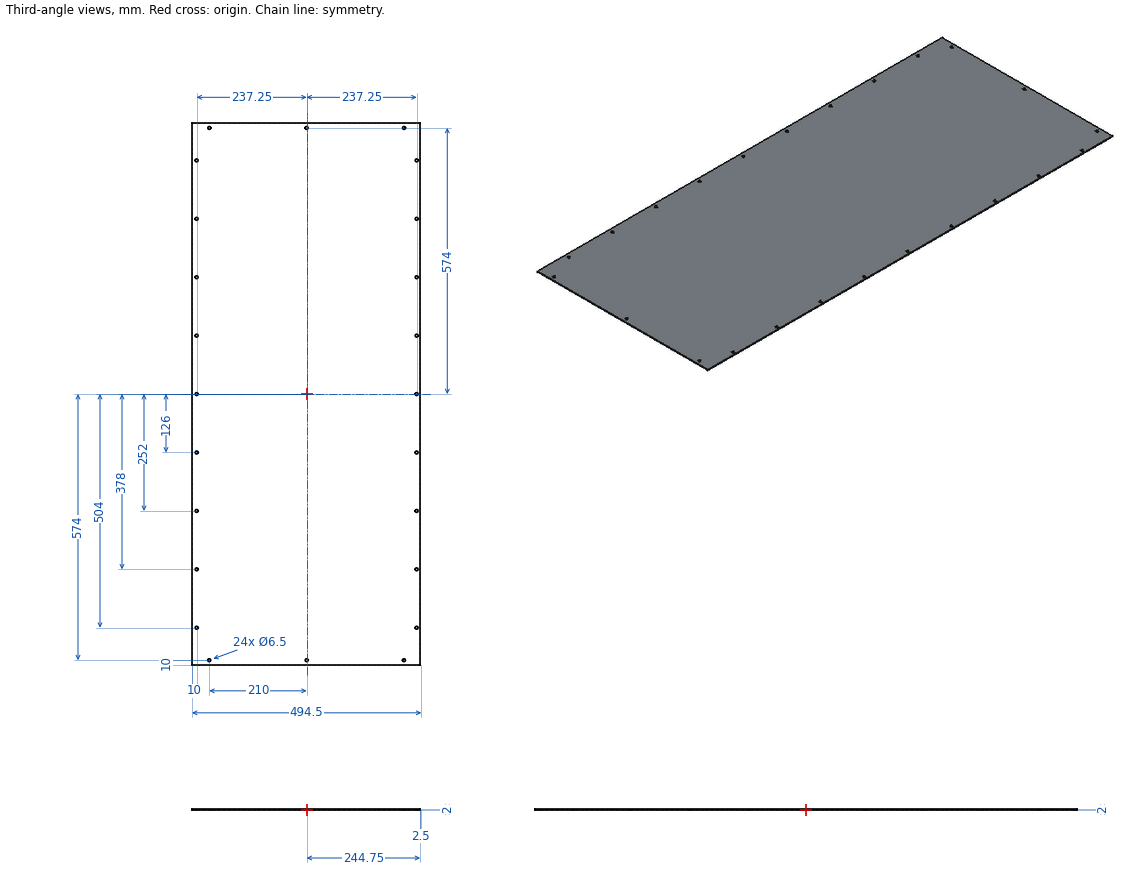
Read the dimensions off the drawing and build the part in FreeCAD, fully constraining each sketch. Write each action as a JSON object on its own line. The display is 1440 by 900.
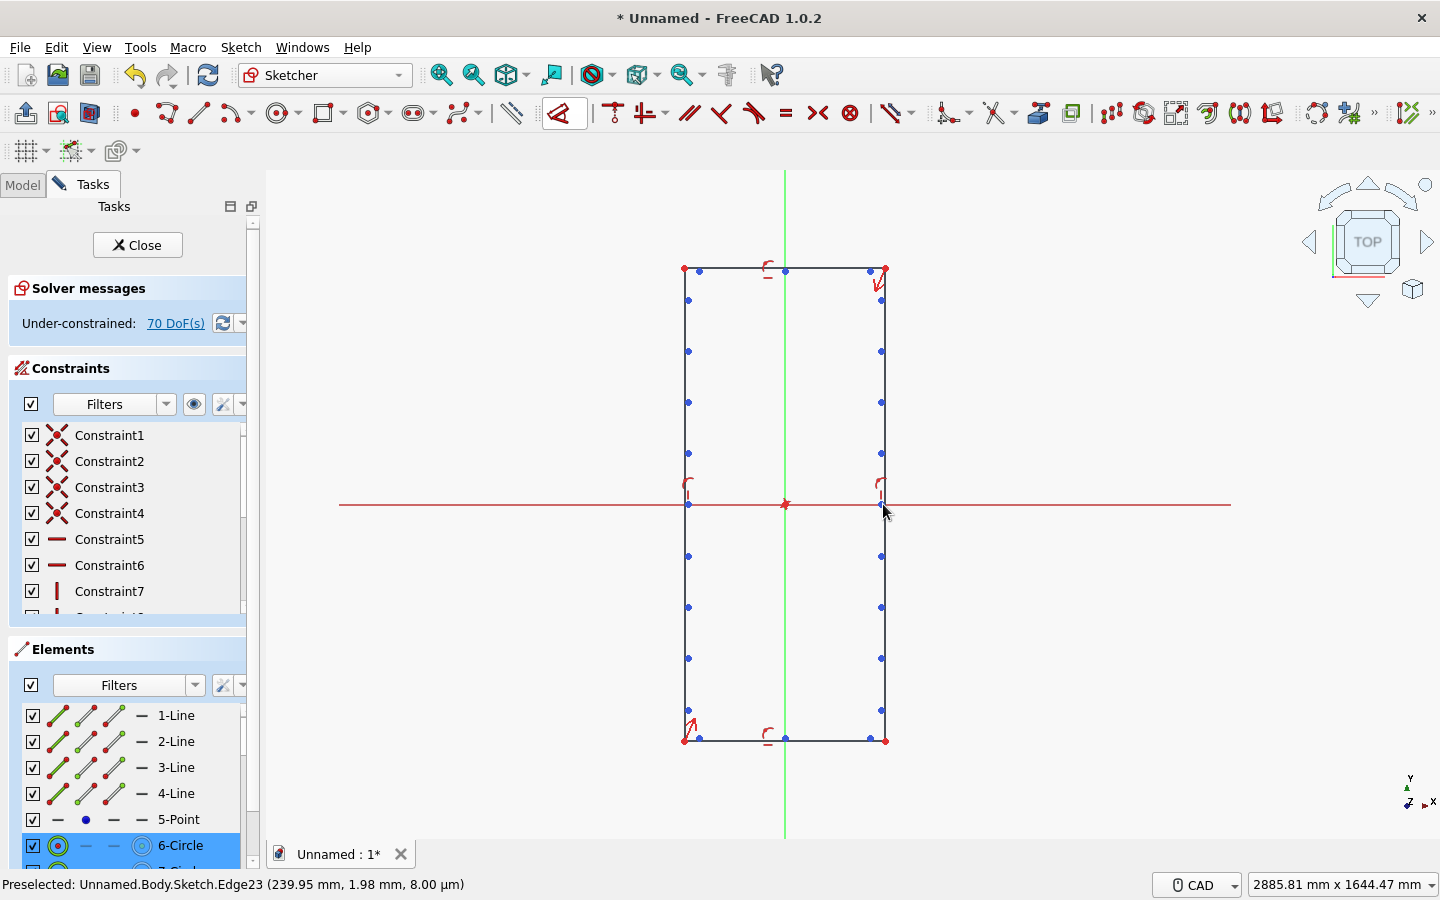
{"action": "scroll", "coordinate": [883, 453], "scroll_direction": "up", "scroll_amount": 12}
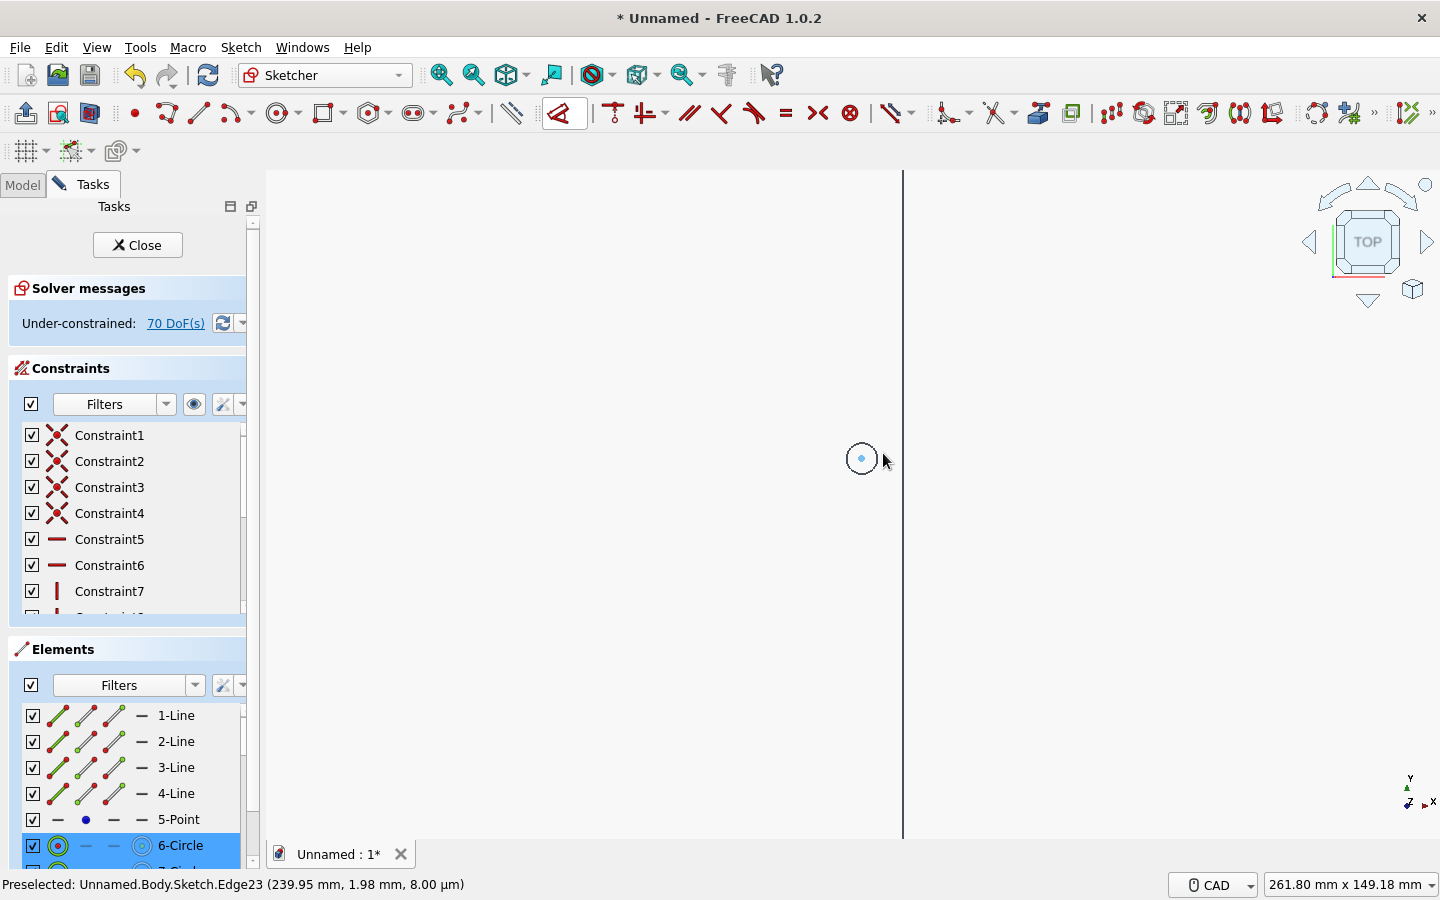
{"action": "left_click", "coordinate": [873, 448]}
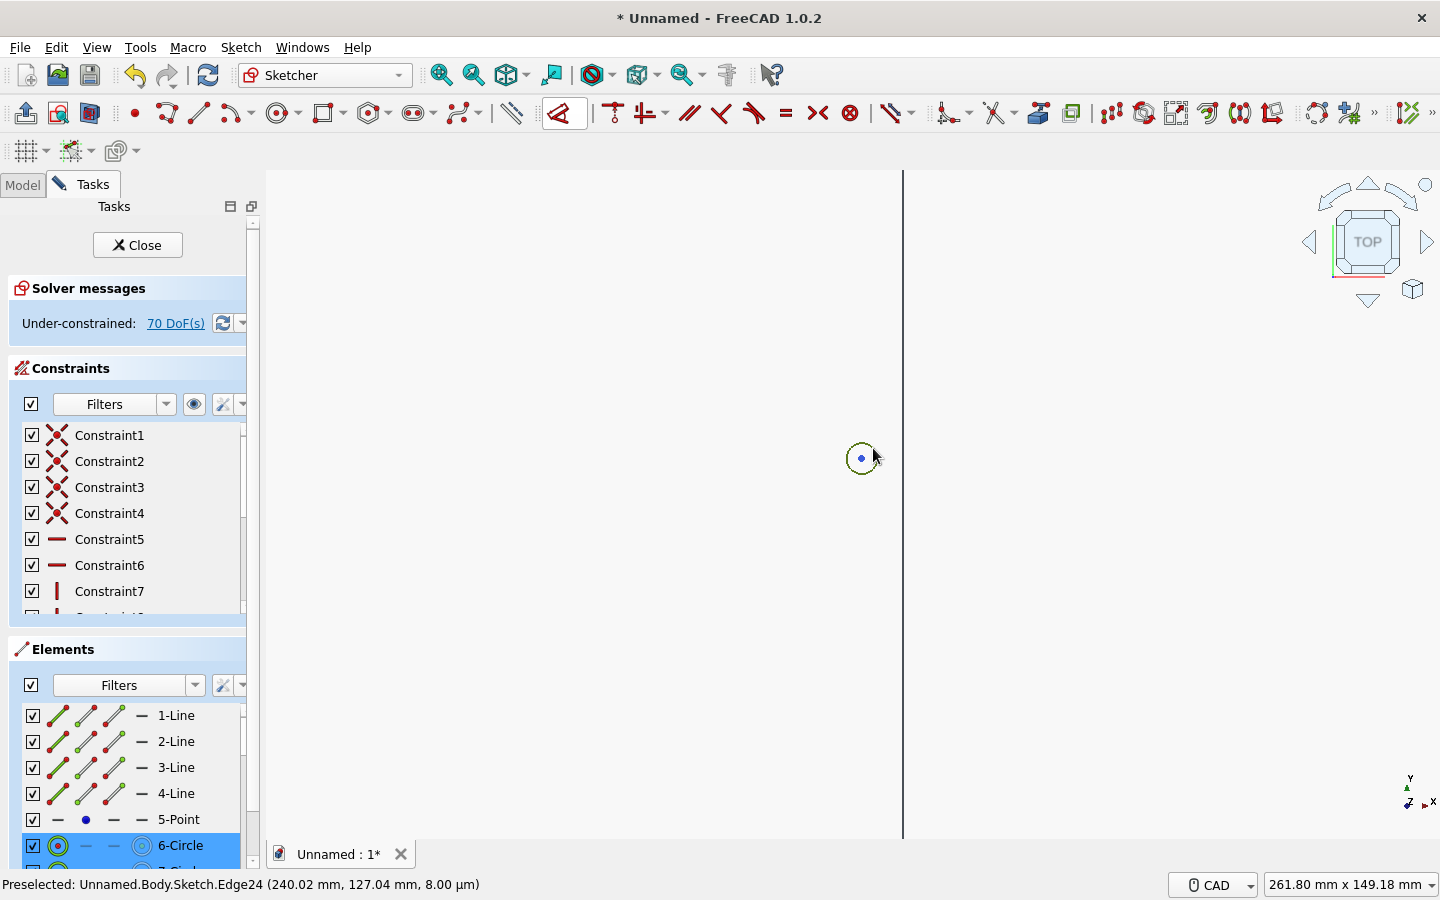
{"action": "scroll", "coordinate": [883, 453], "scroll_direction": "down", "scroll_amount": 12}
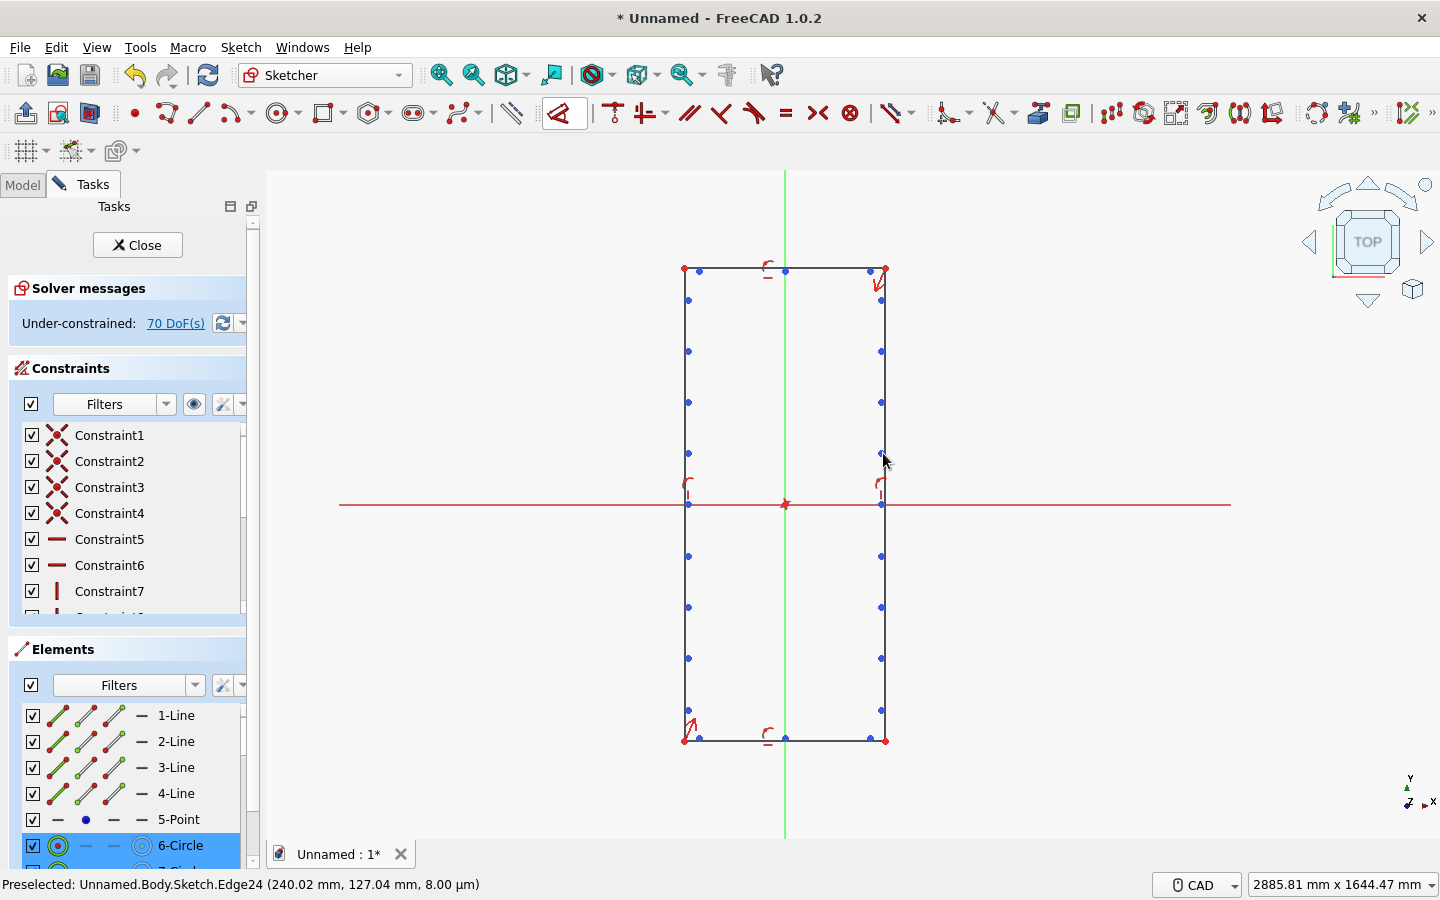
{"action": "scroll", "coordinate": [883, 402], "scroll_direction": "up", "scroll_amount": 12}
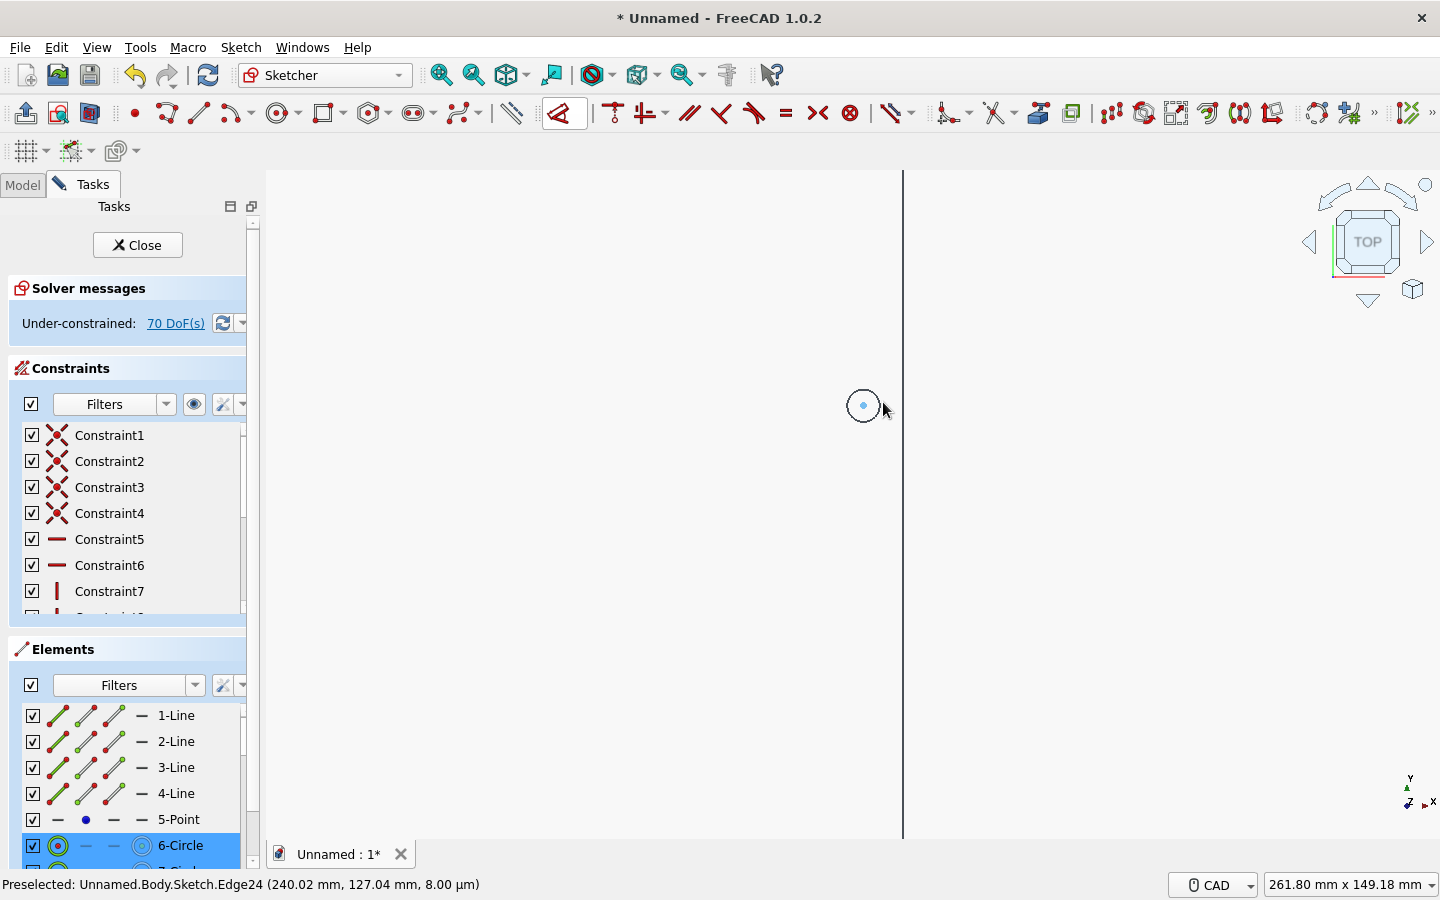
{"action": "left_click", "coordinate": [875, 394]}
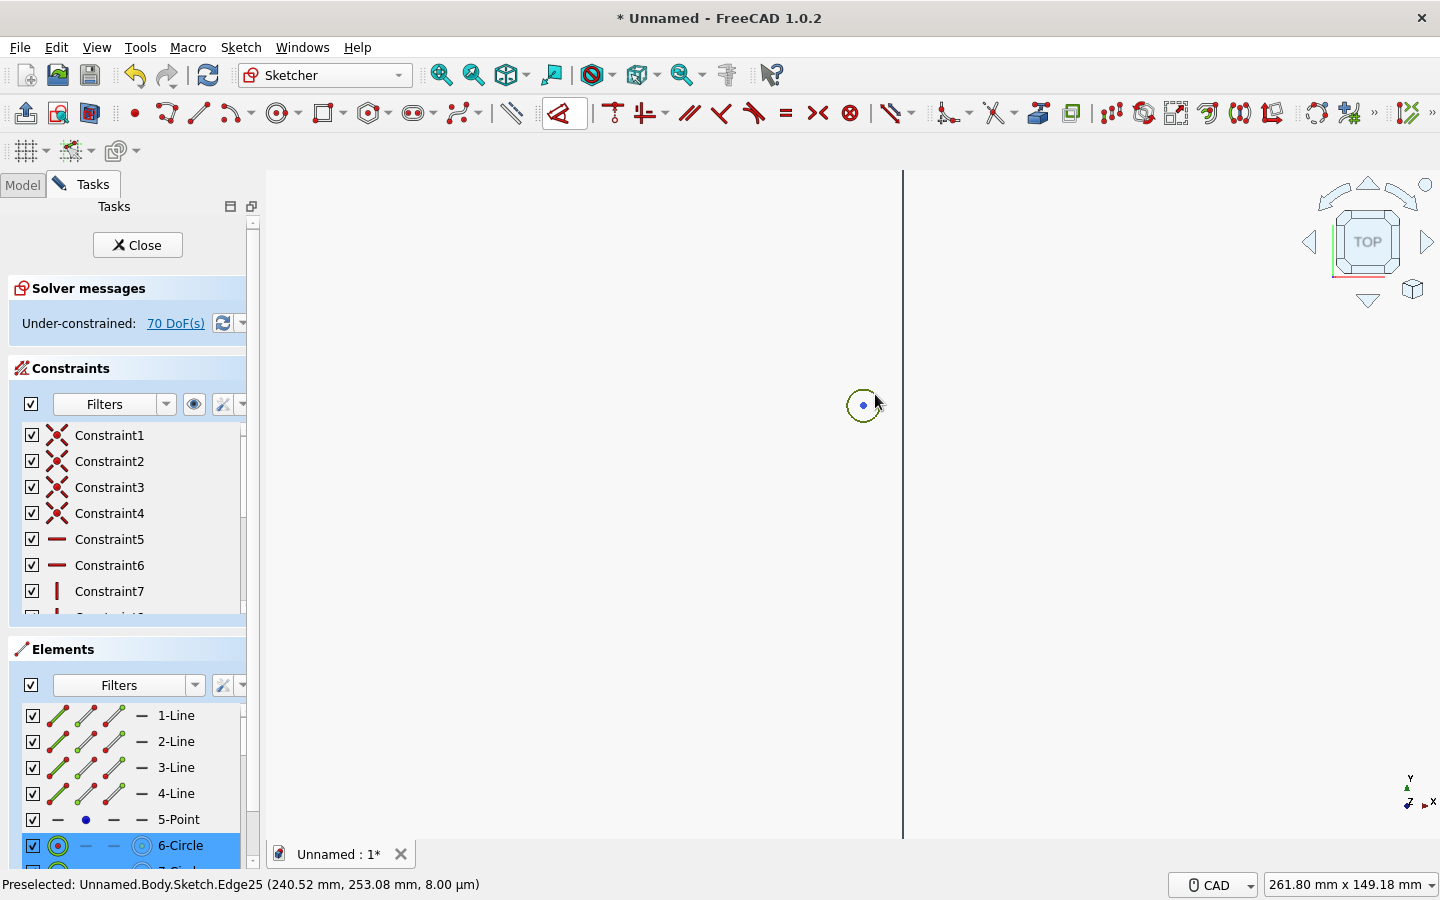
{"action": "scroll", "coordinate": [883, 402], "scroll_direction": "down", "scroll_amount": 12}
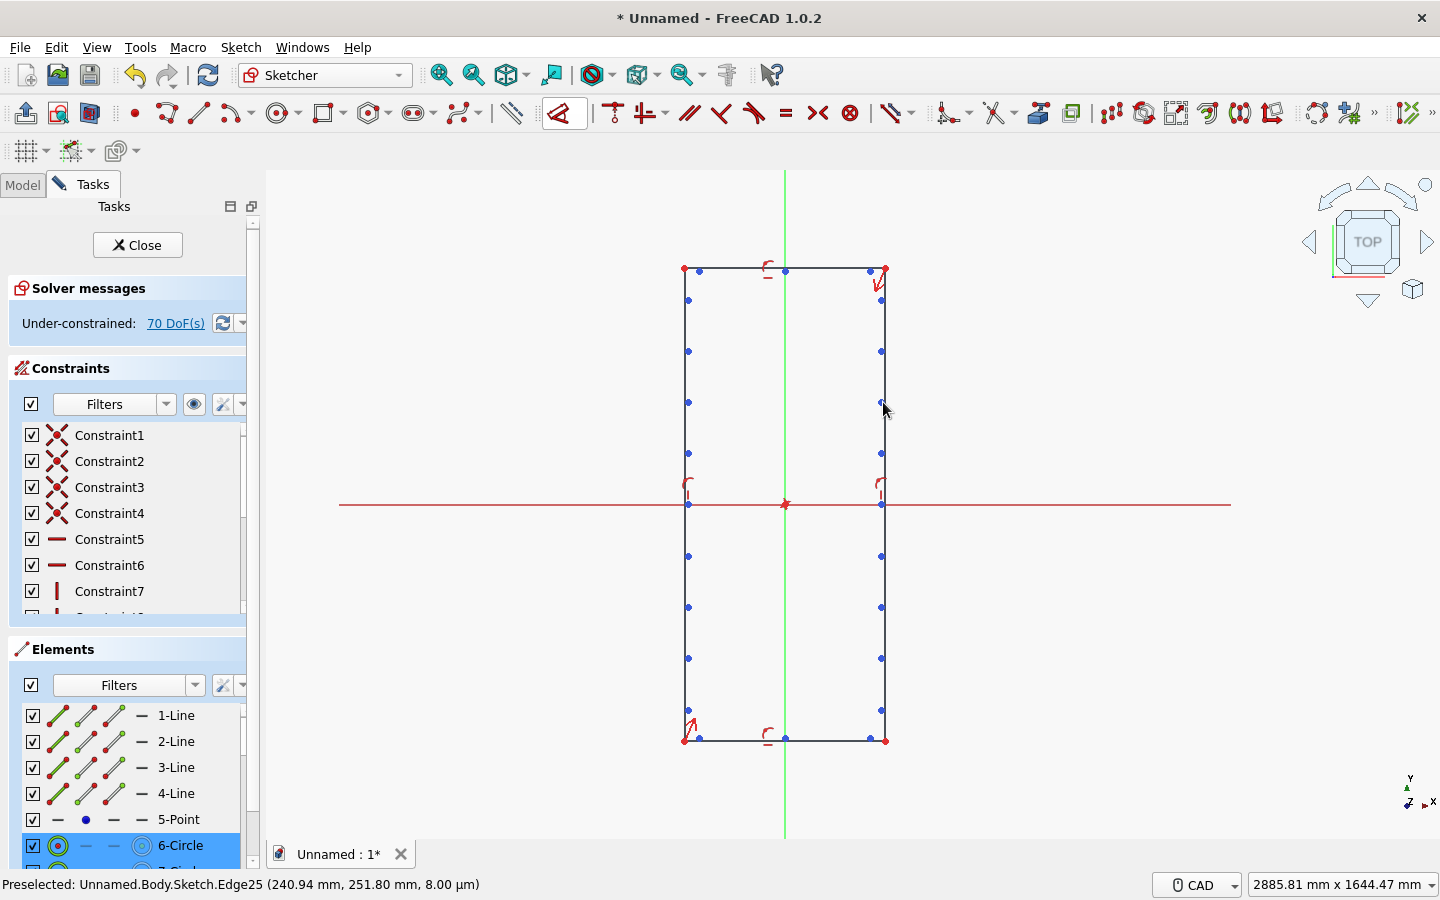
{"action": "scroll", "coordinate": [786, 271], "scroll_direction": "up", "scroll_amount": 14}